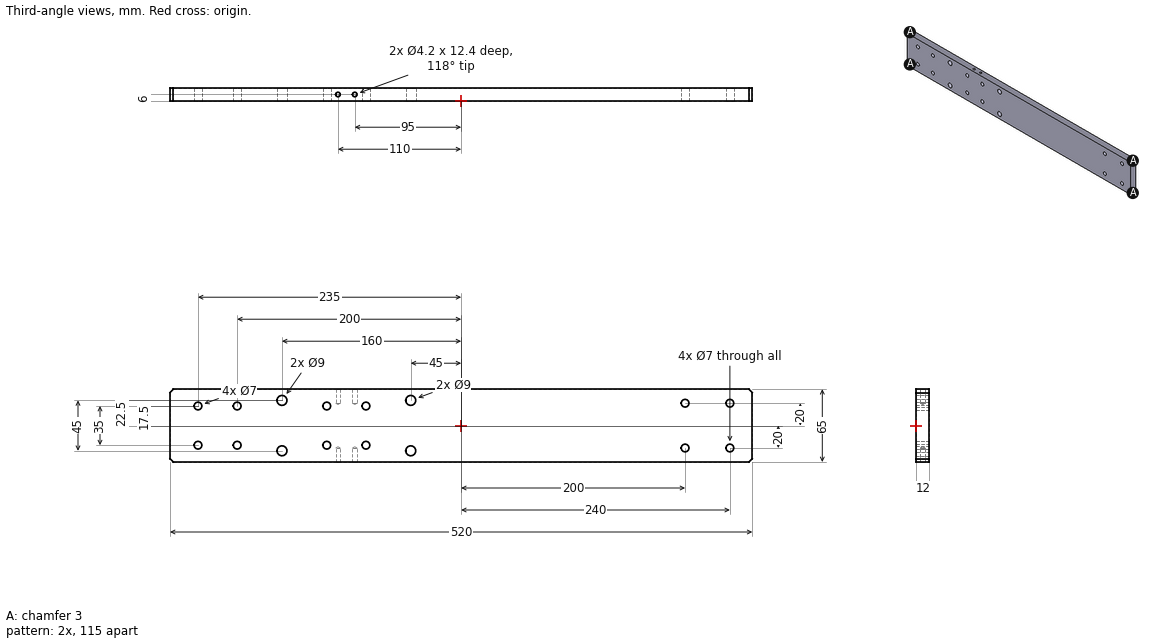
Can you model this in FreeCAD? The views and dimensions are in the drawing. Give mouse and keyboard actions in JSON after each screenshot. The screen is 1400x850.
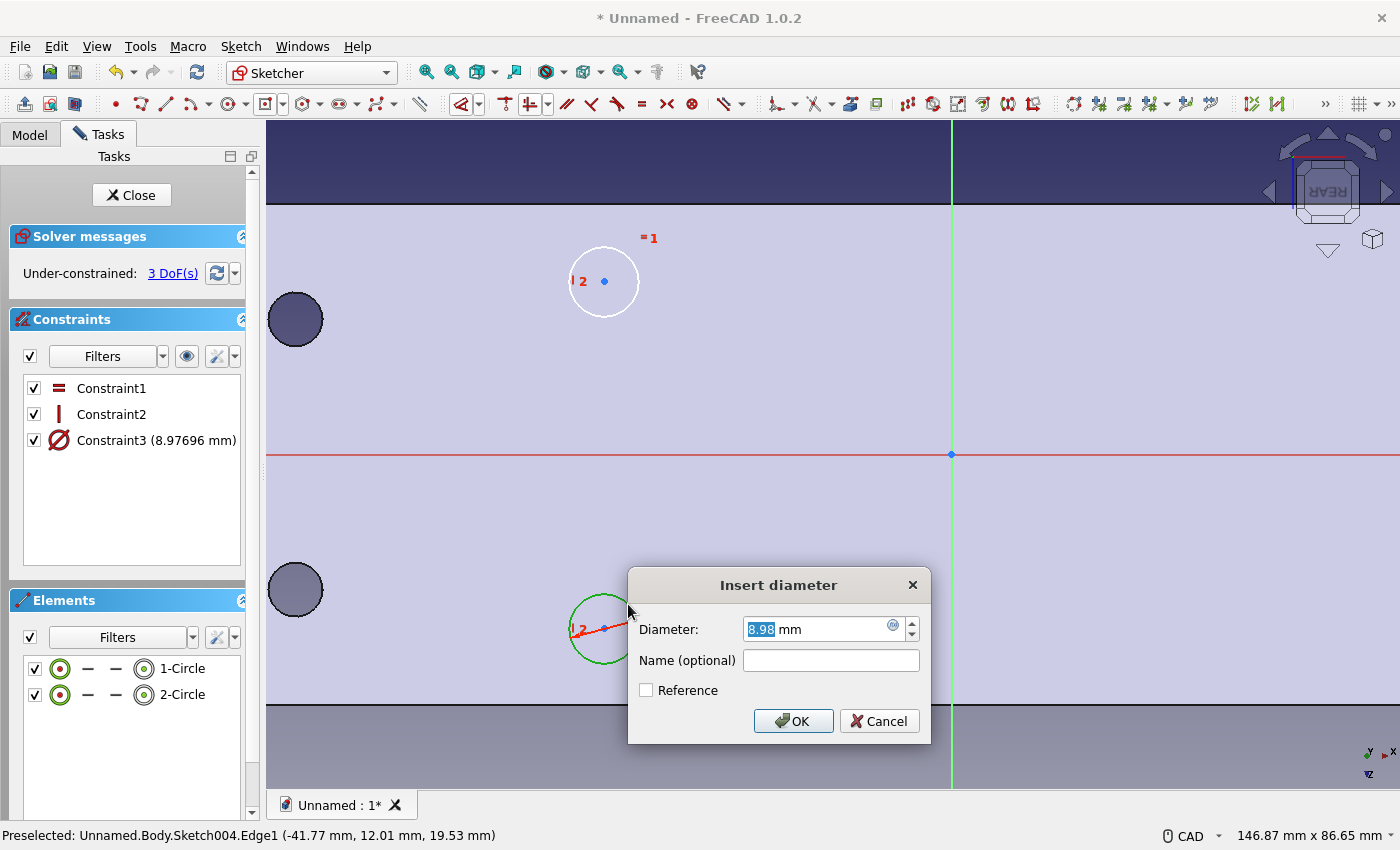
{"action": "type", "text": "9"}
{"action": "key", "text": "Return"}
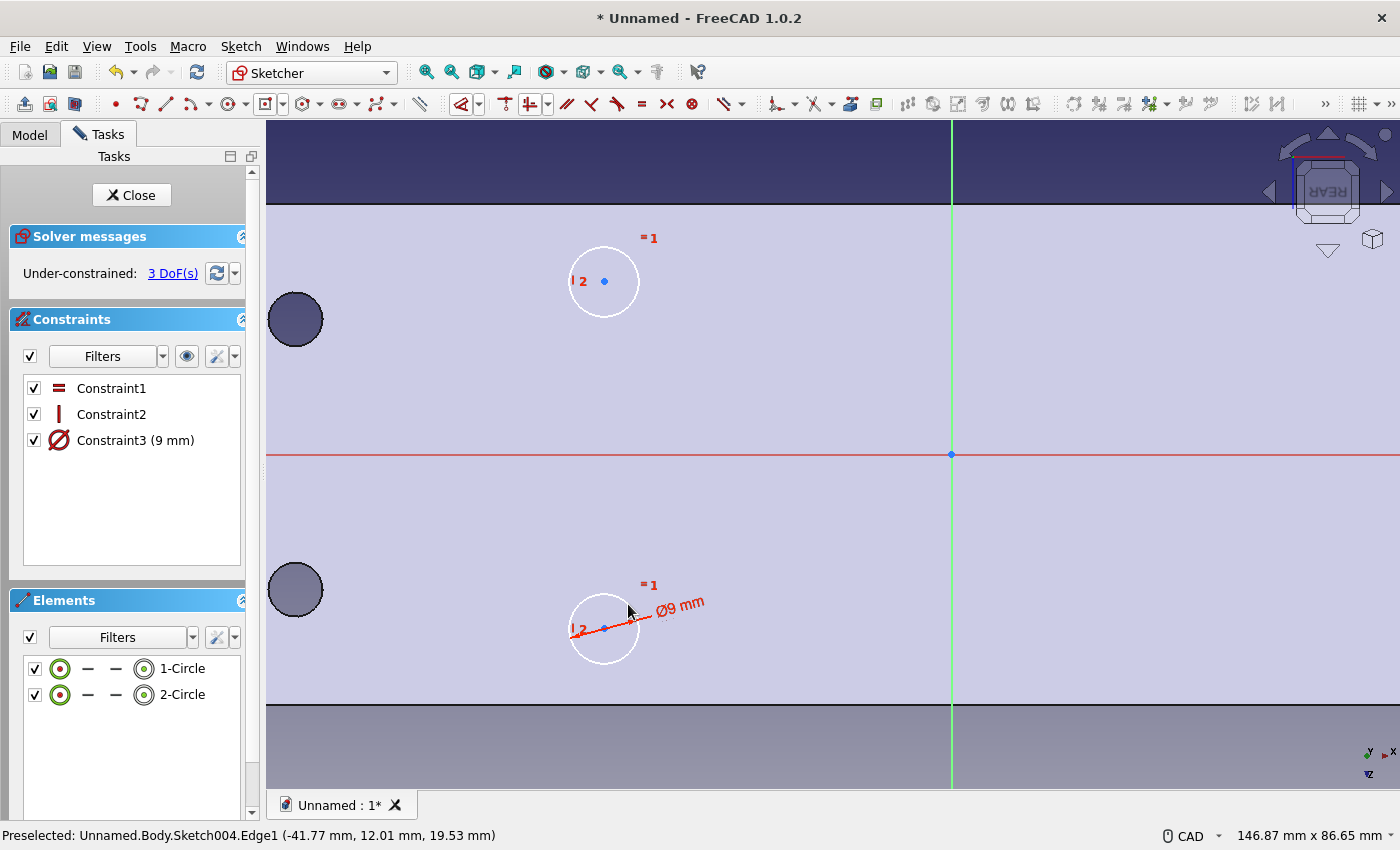
{"action": "left_click", "coordinate": [604, 629]}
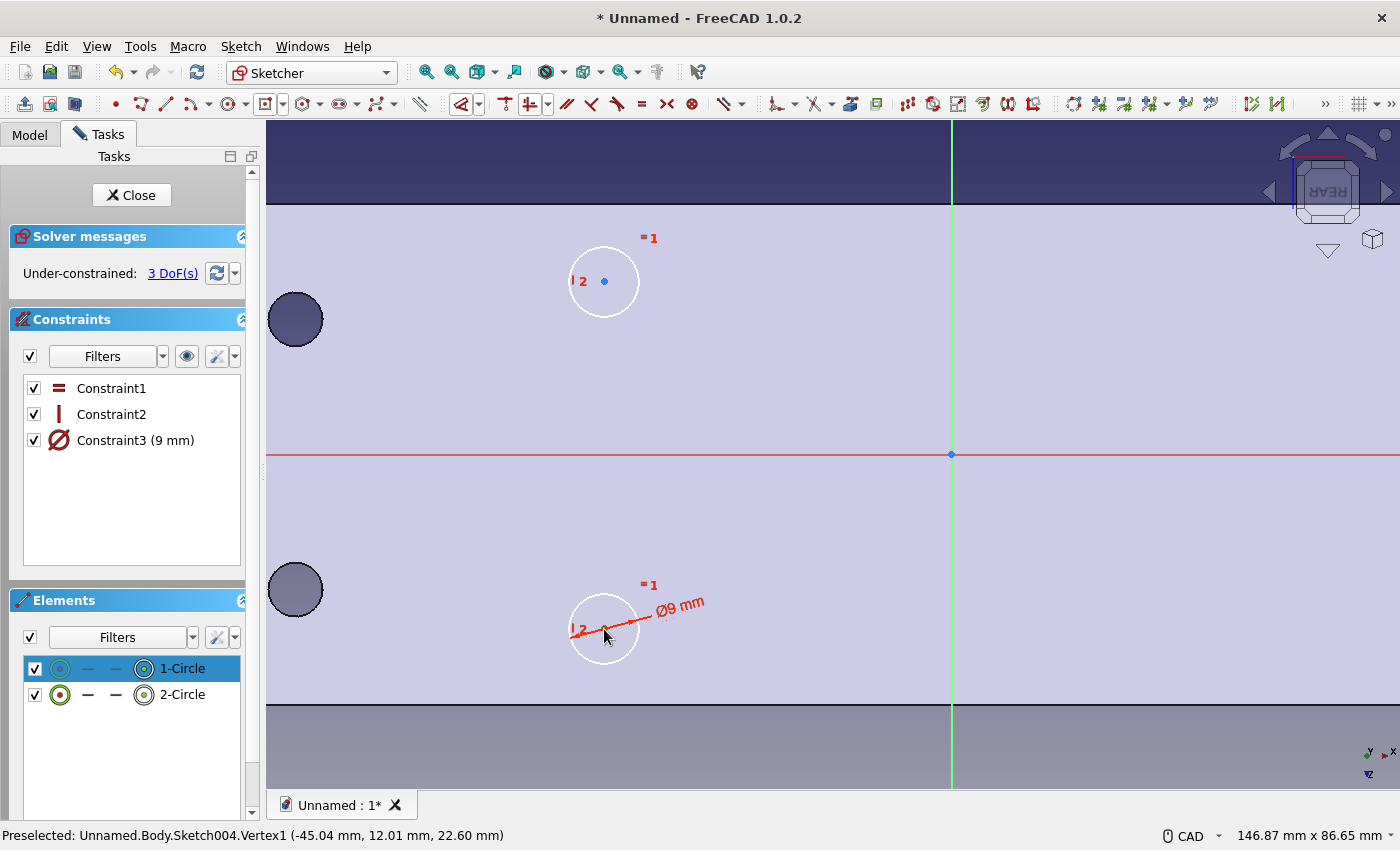
{"action": "key", "text": "l"}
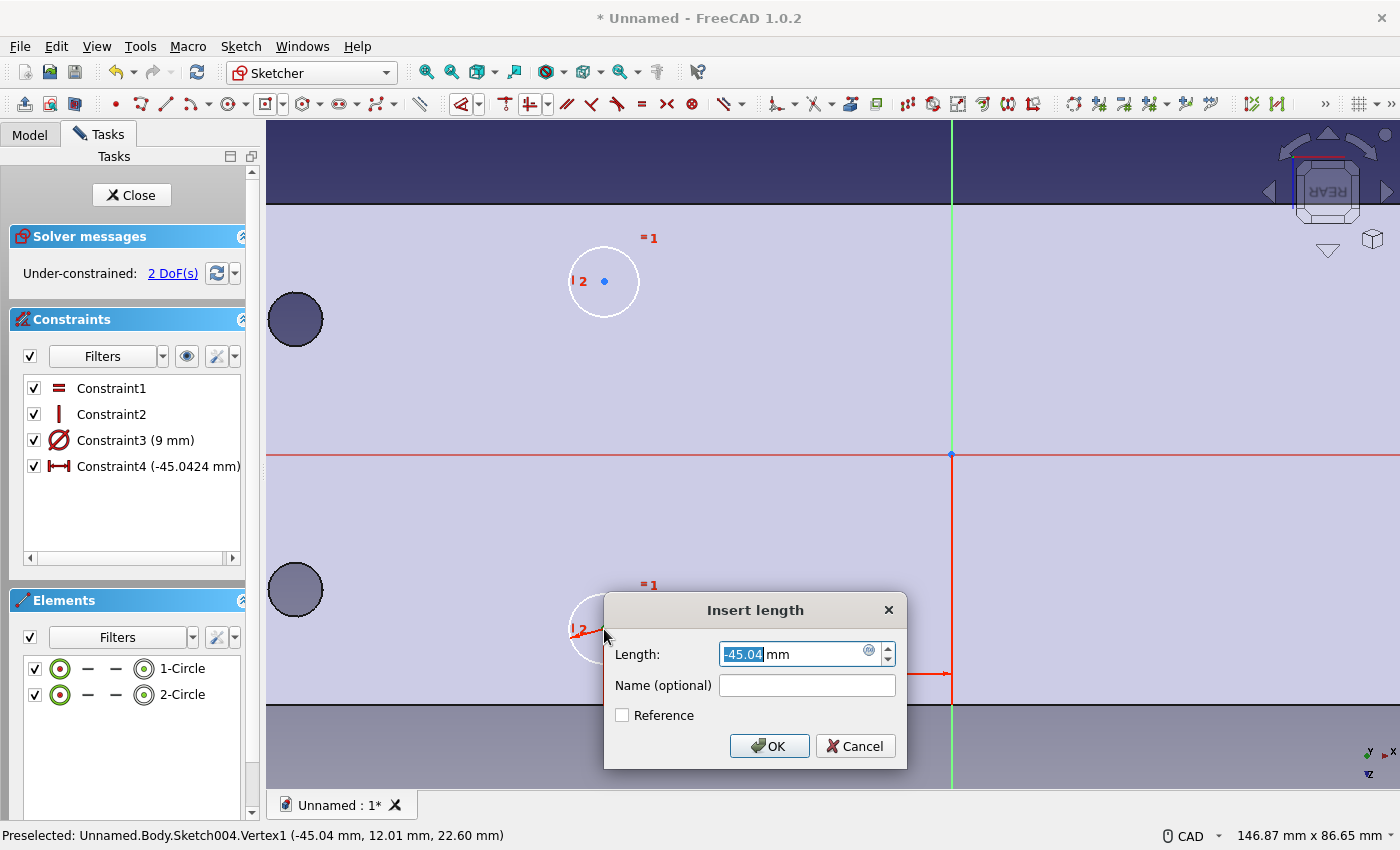
{"action": "type", "text": "-45"}
{"action": "key", "text": "Return"}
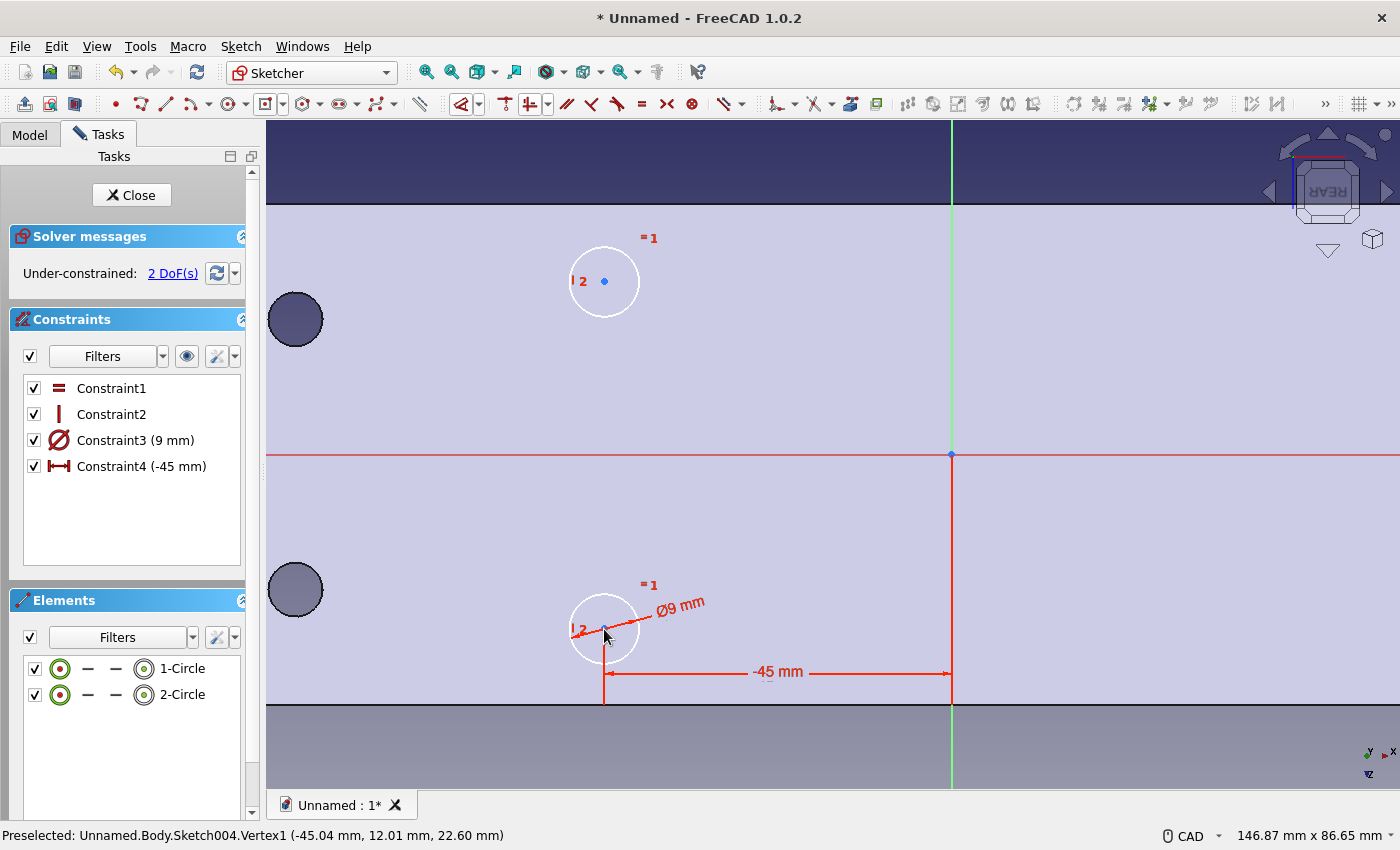
{"action": "left_click", "coordinate": [604, 629]}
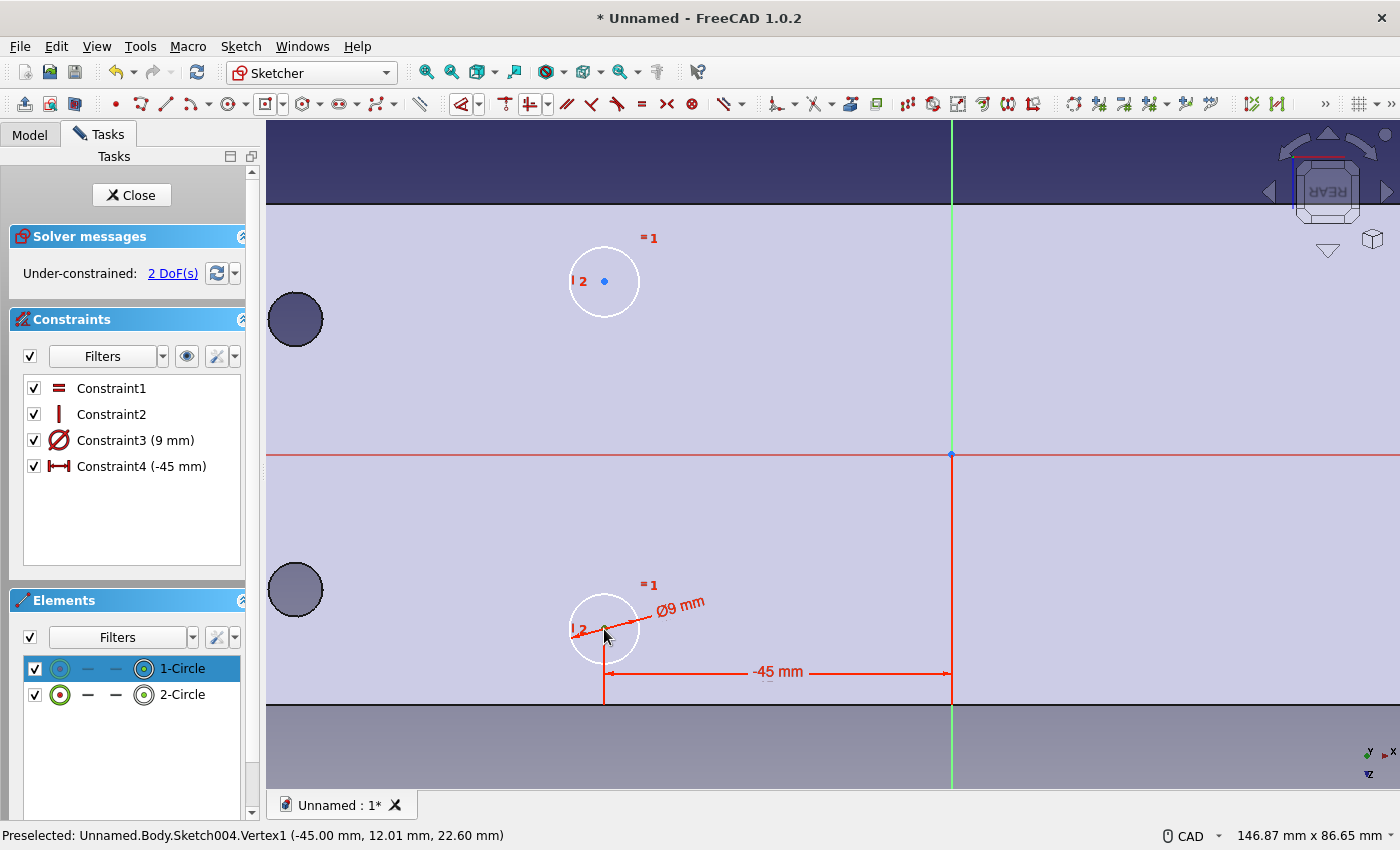
{"action": "left_click", "coordinate": [604, 282]}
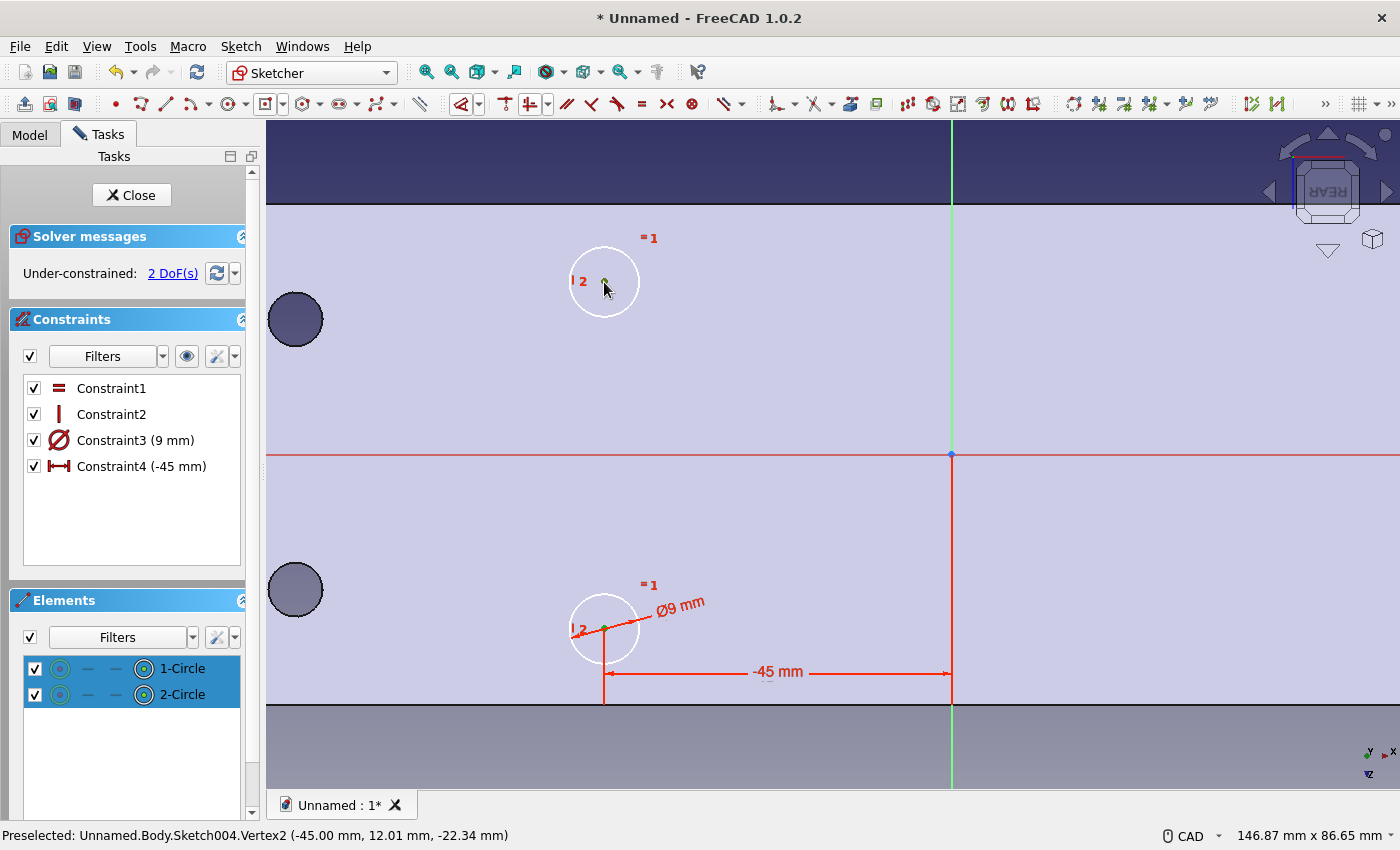
{"action": "key", "text": "i"}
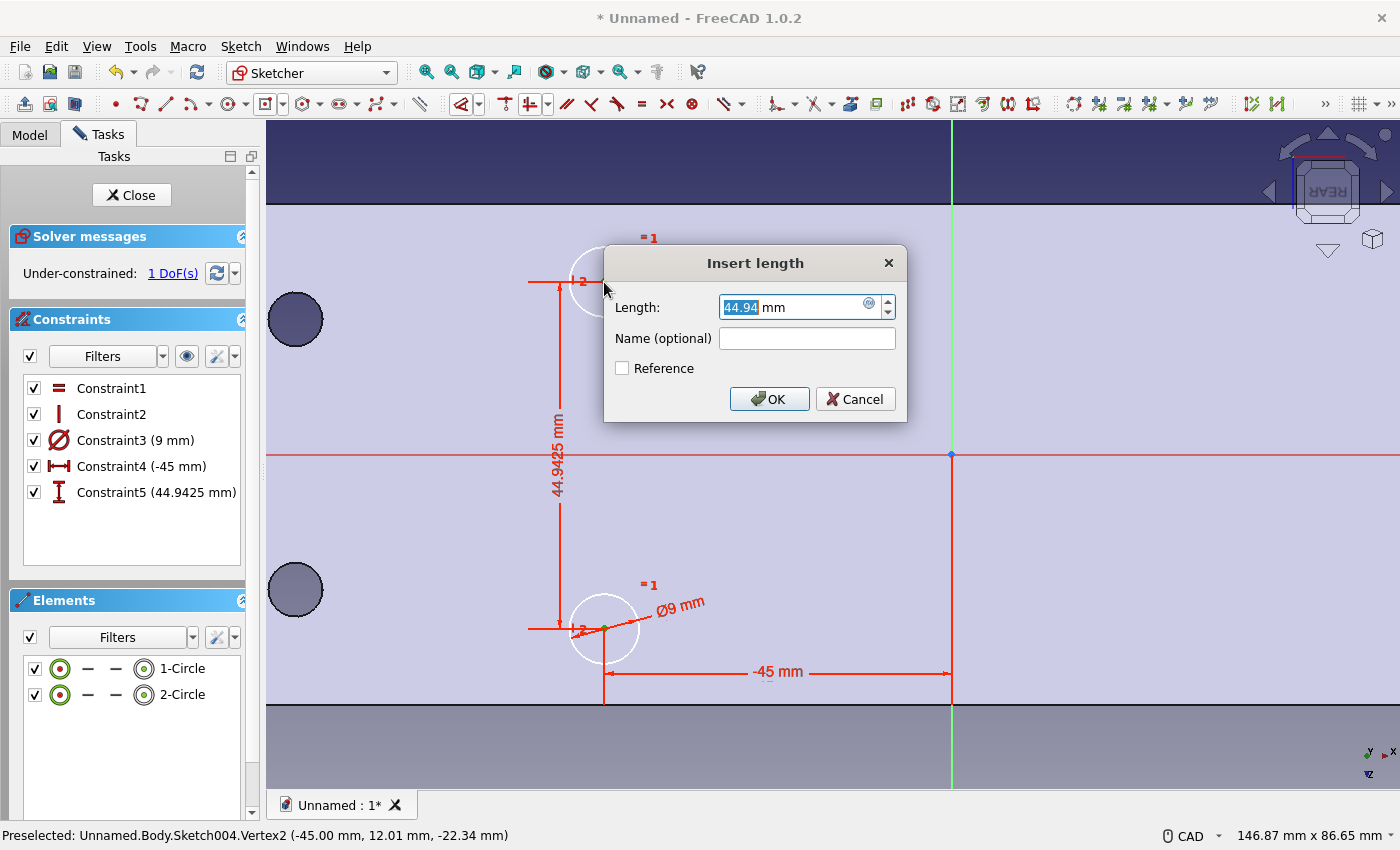
{"action": "type", "text": "45"}
{"action": "key", "text": "Return"}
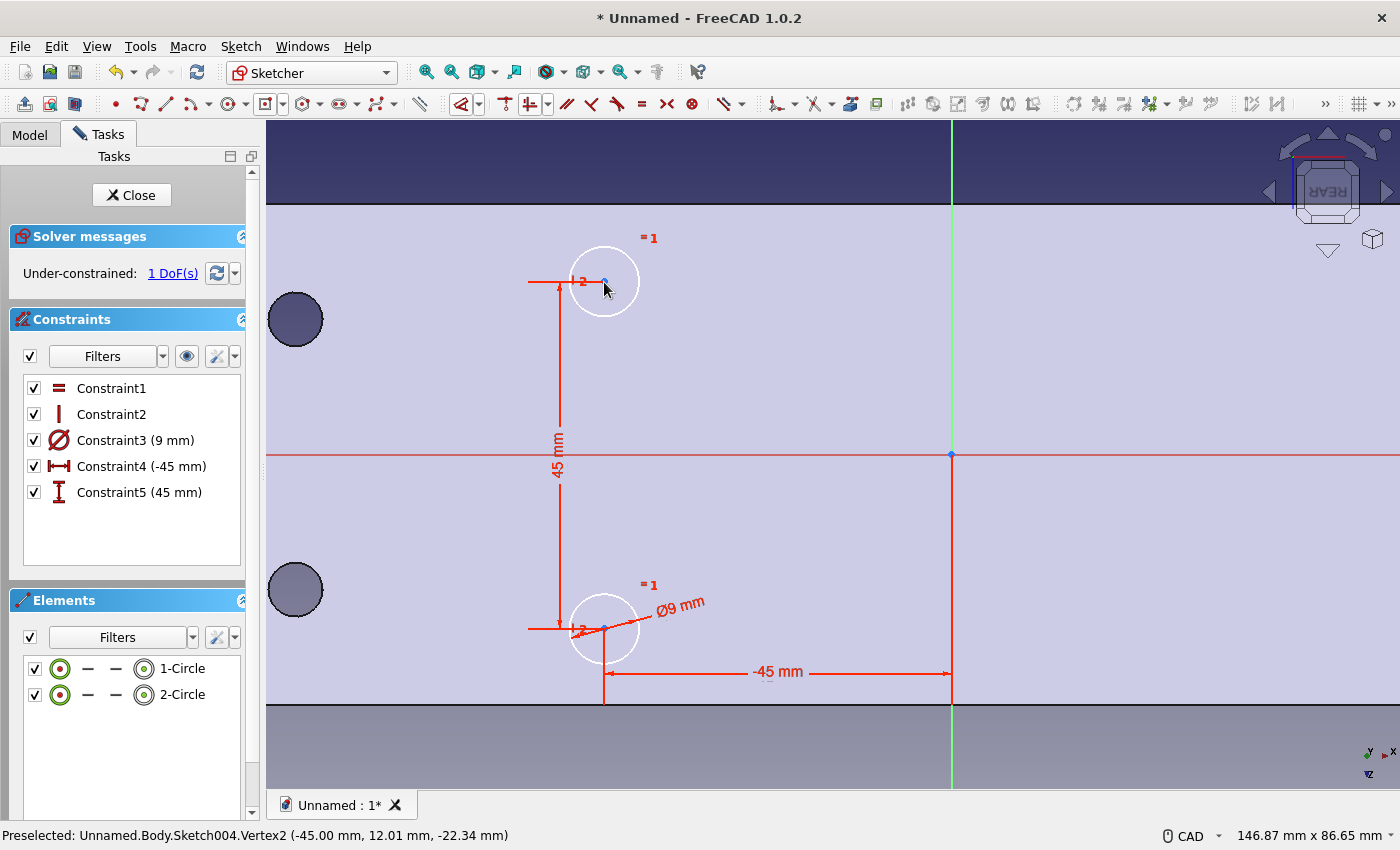
{"action": "left_click", "coordinate": [604, 629]}